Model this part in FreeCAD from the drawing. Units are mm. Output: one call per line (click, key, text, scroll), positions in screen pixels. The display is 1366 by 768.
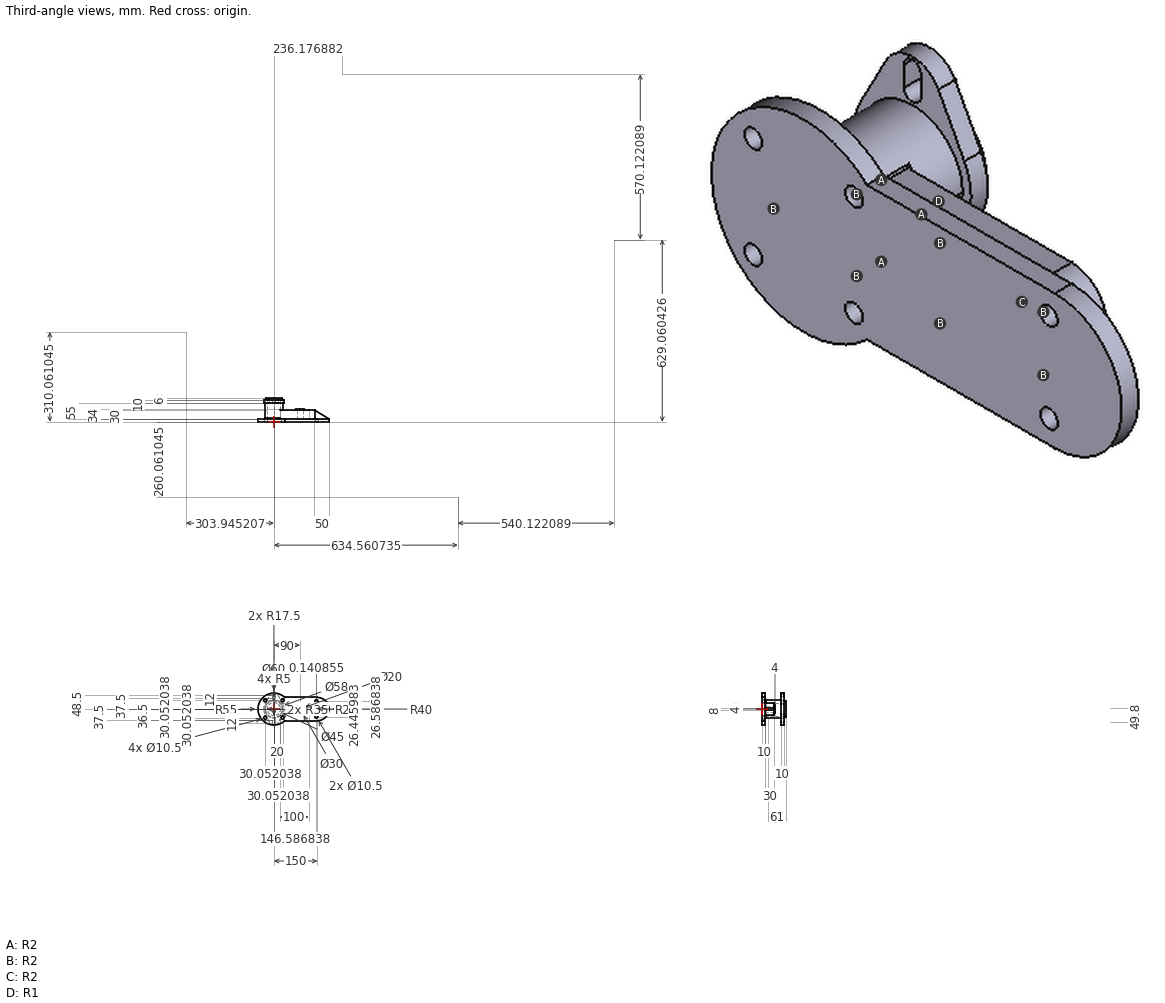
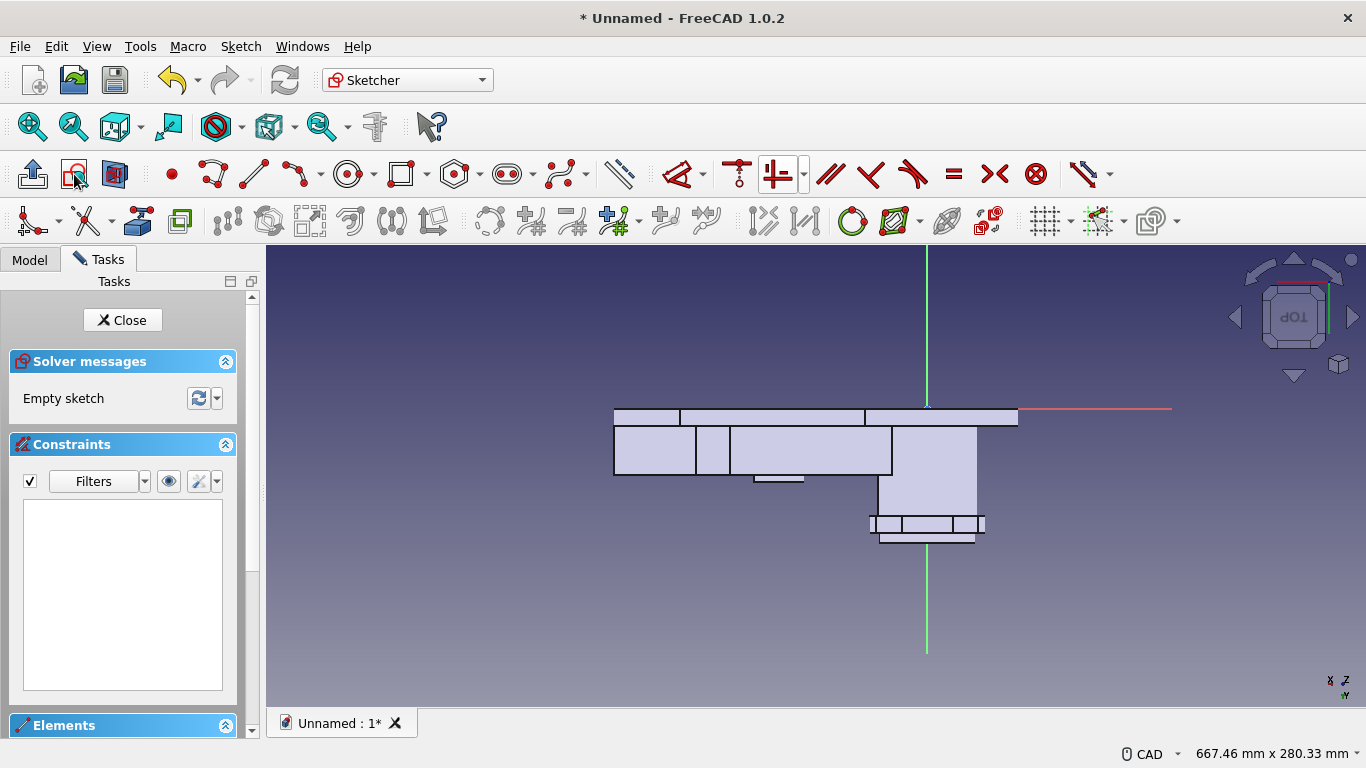
key(q)
key(s)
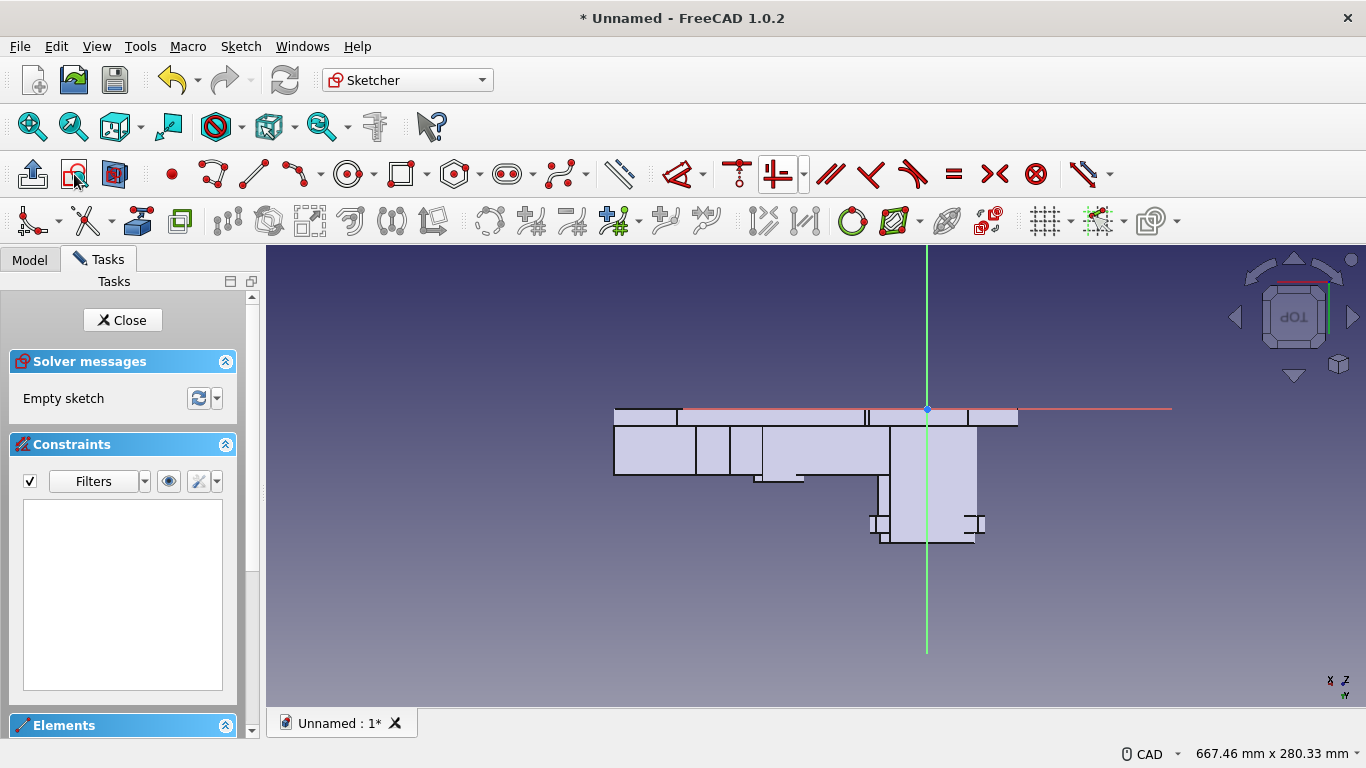
scroll(814, 388, down, 11)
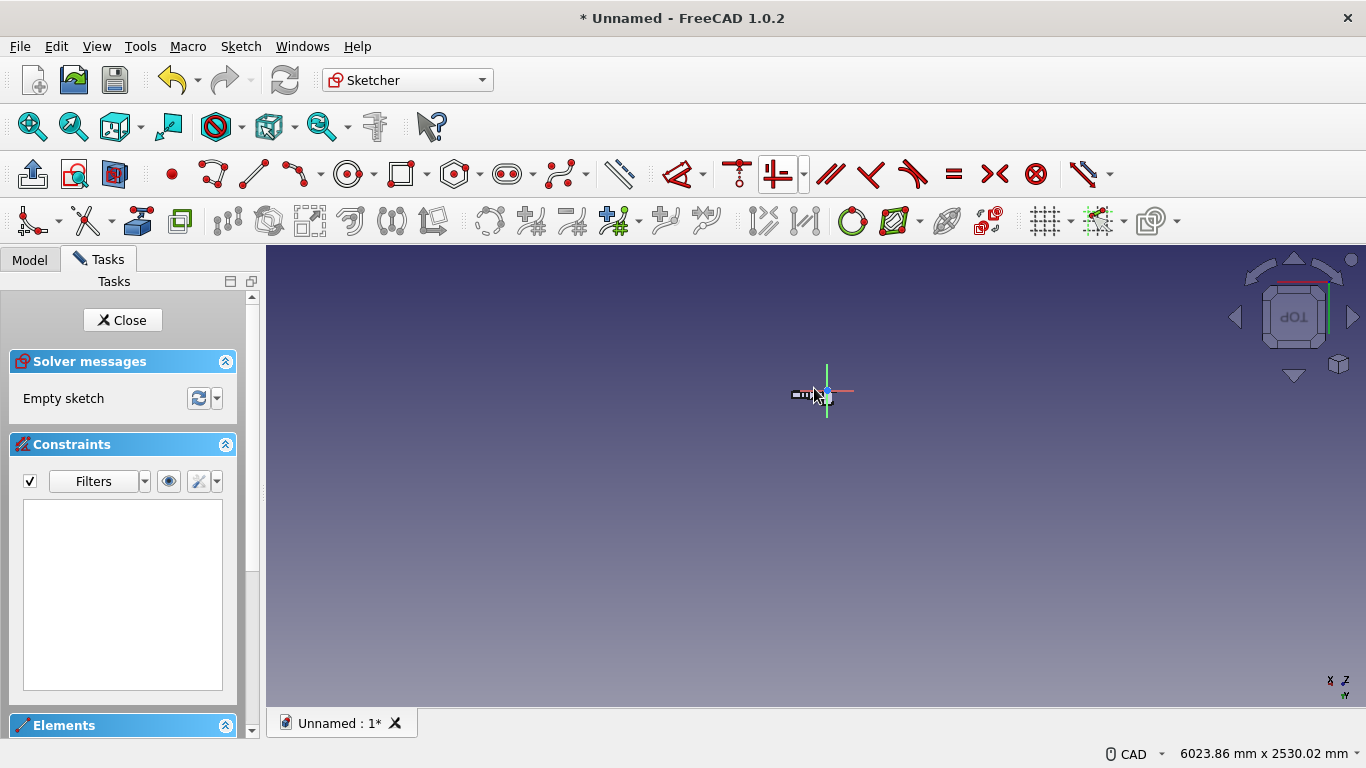
click(213, 174)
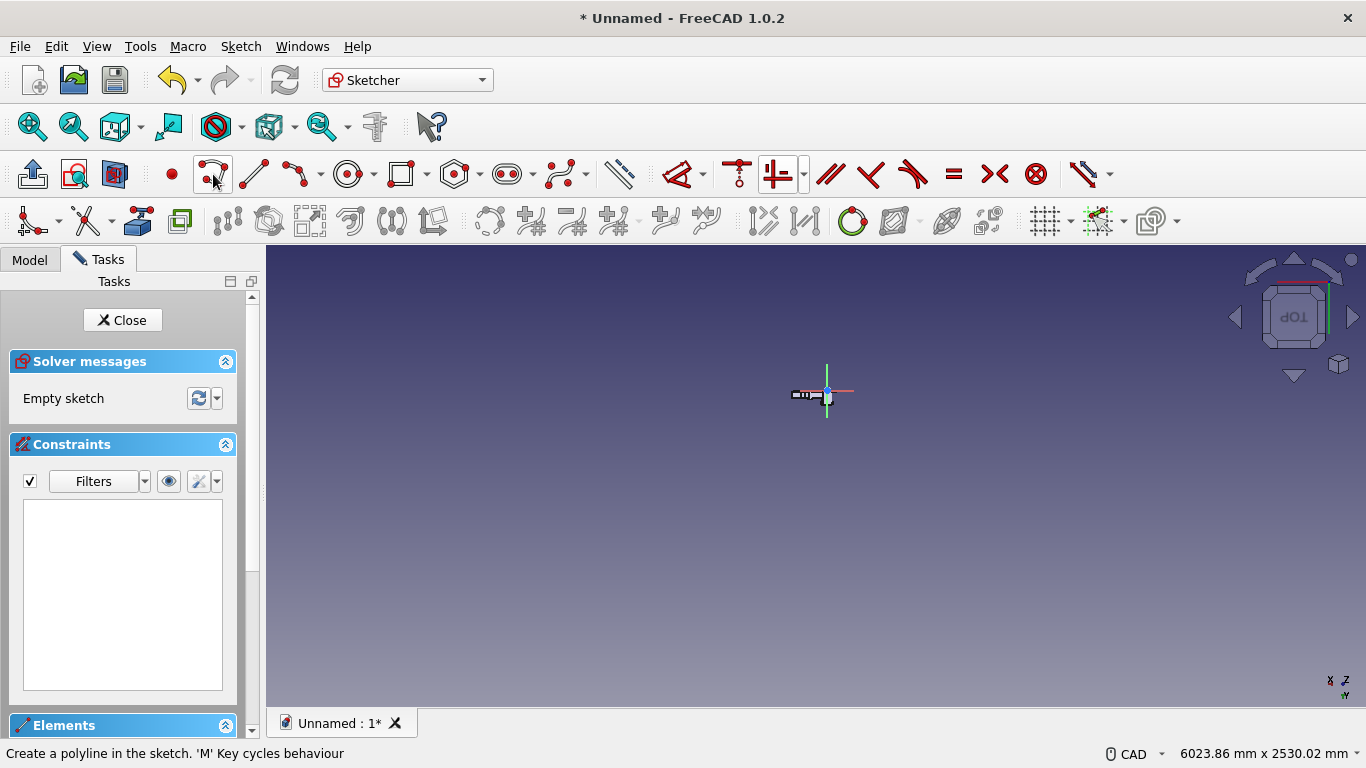
click(883, 447)
click(711, 343)
click(612, 506)
click(784, 610)
click(883, 448)
key(Escape)
key(Escape)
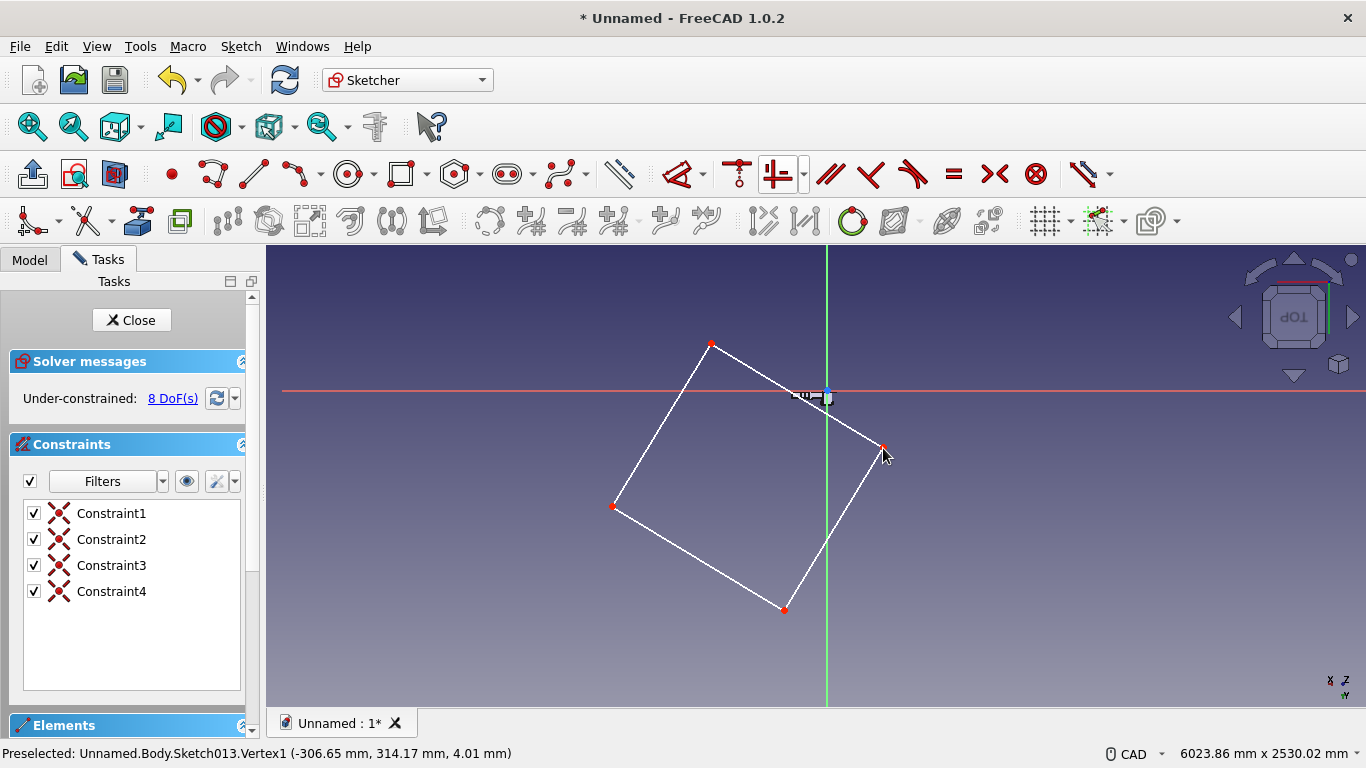
key(d)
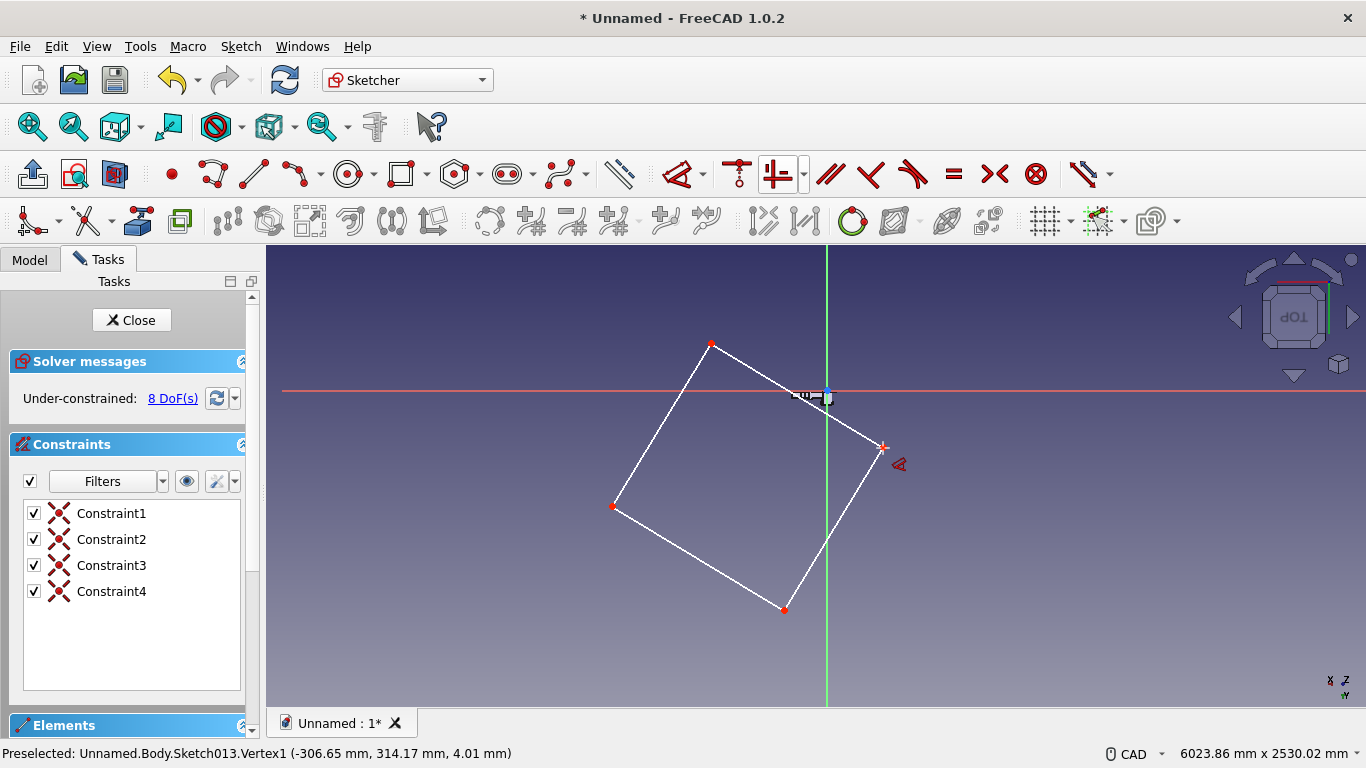
click(883, 448)
click(855, 357)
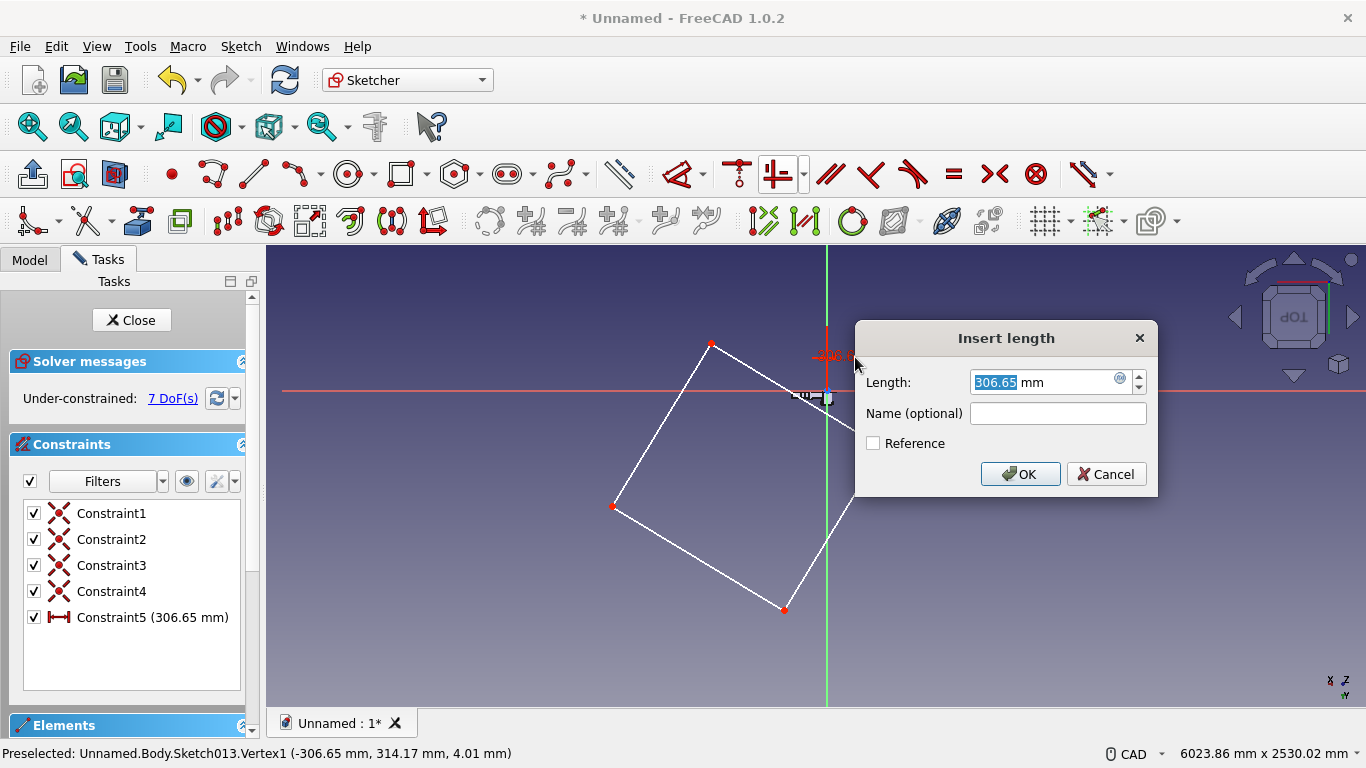
text(303.945207)
key(Return)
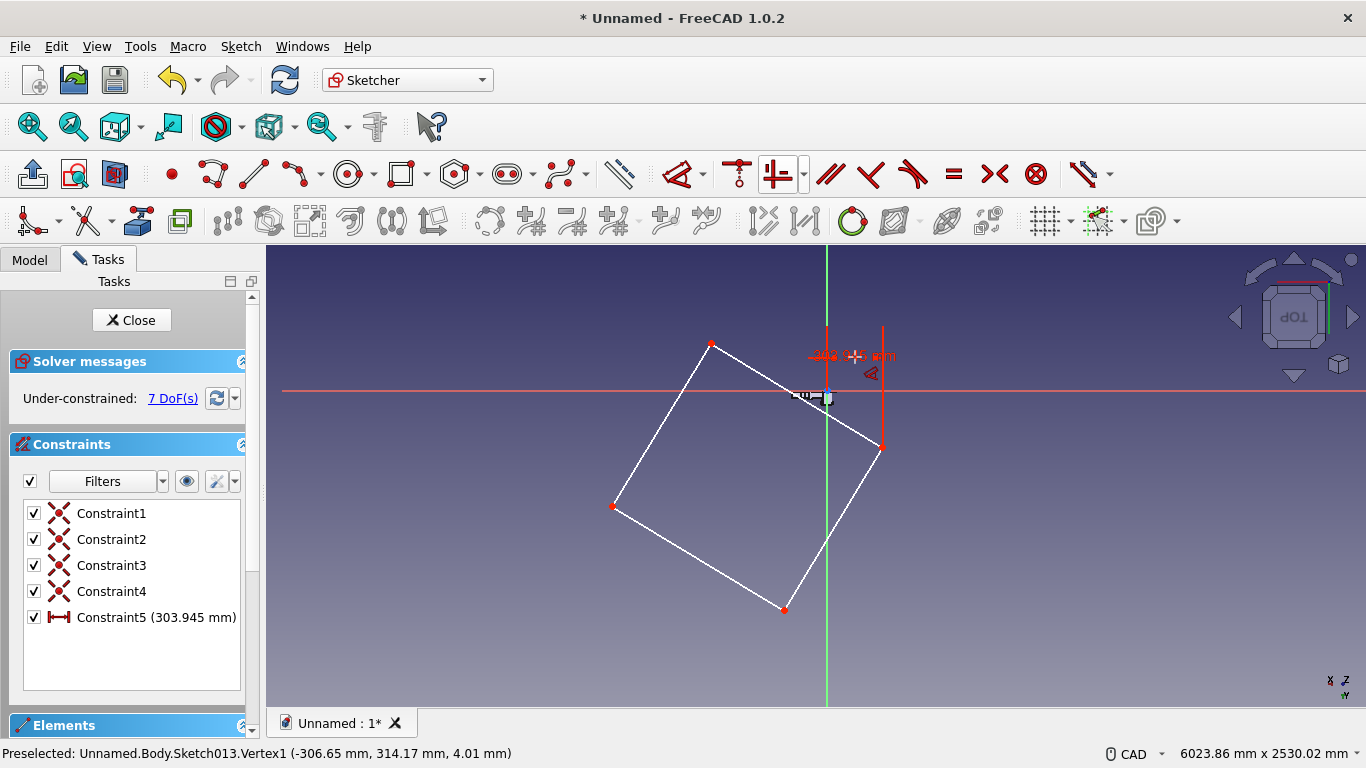
click(883, 448)
click(917, 419)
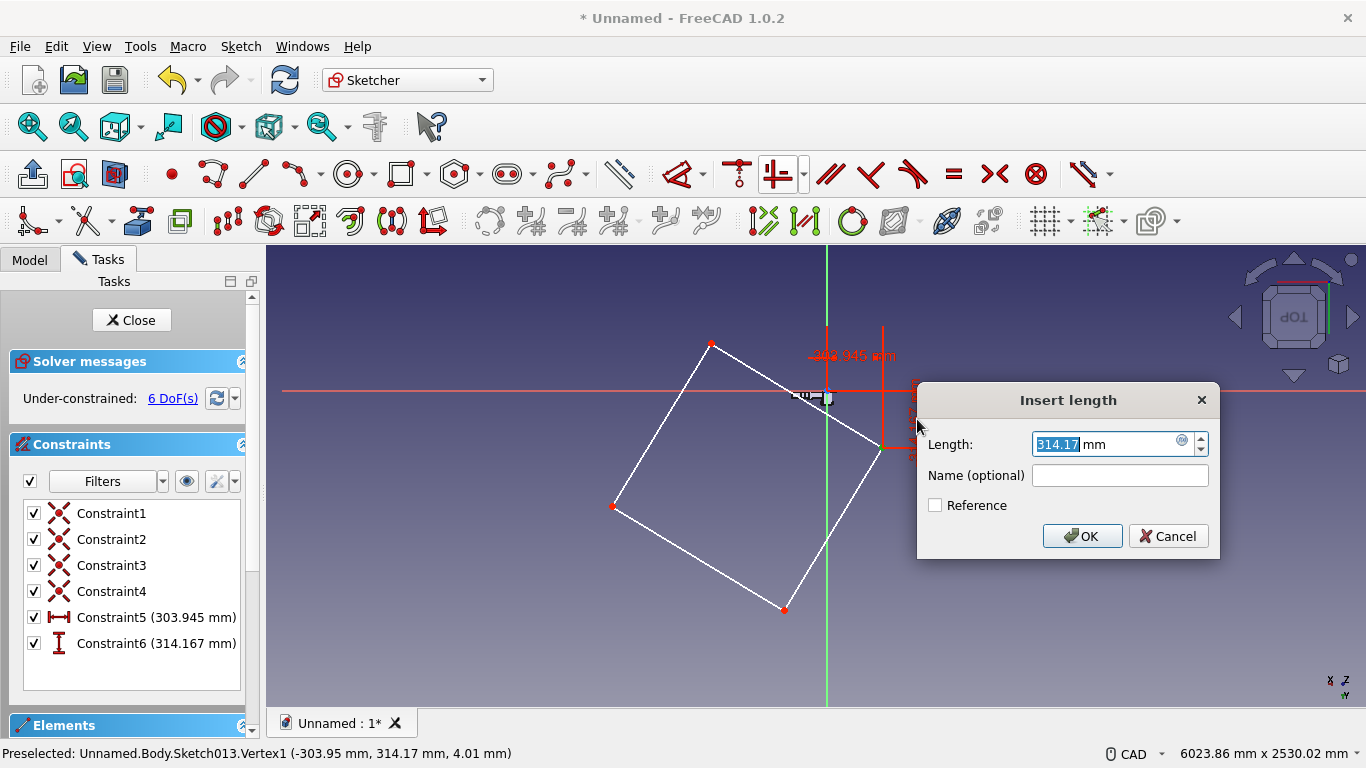
text(310.061045)
key(Return)